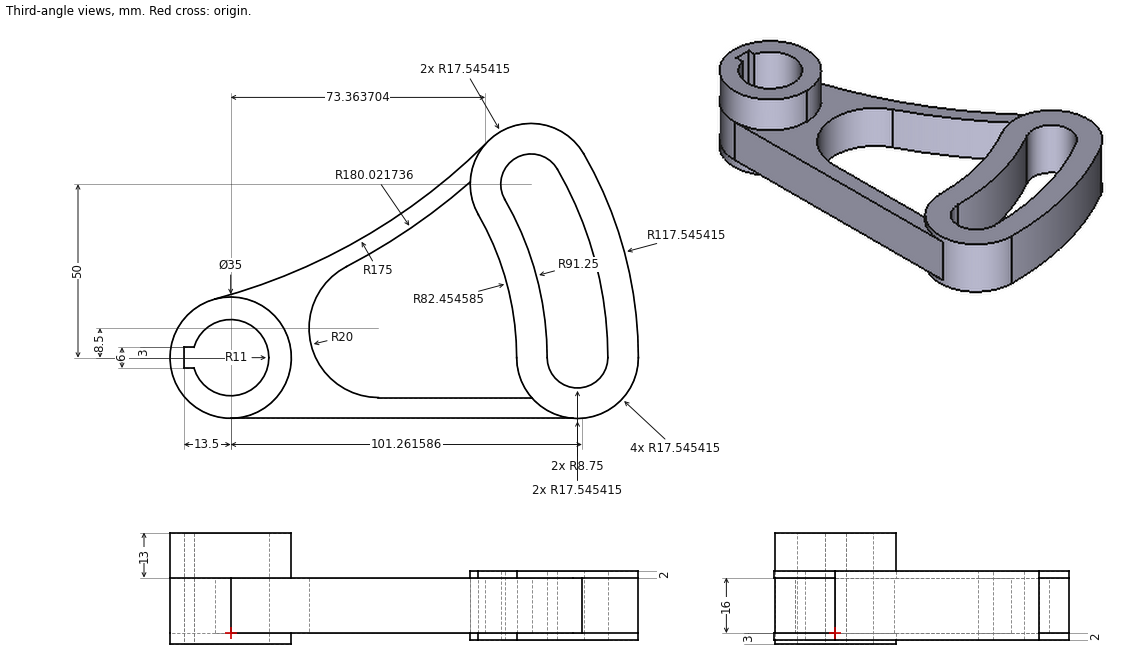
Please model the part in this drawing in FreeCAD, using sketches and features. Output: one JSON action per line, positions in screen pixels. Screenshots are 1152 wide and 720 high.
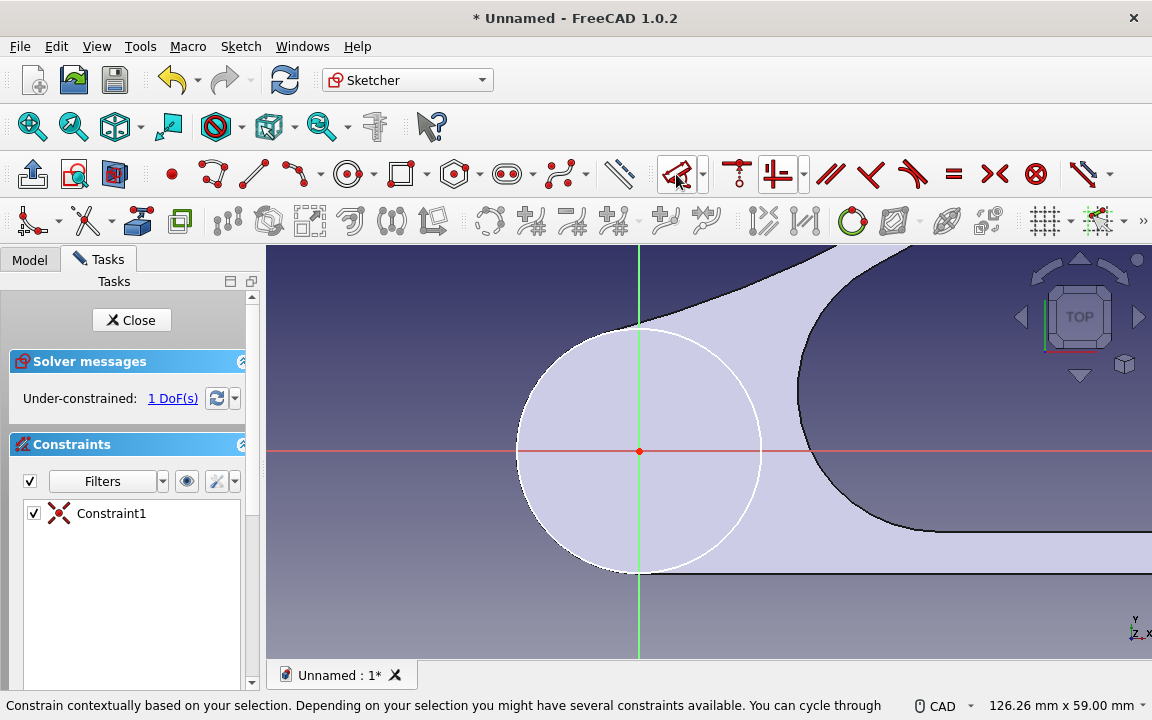
{"action": "left_click", "coordinate": [725, 364]}
{"action": "left_click", "coordinate": [747, 341]}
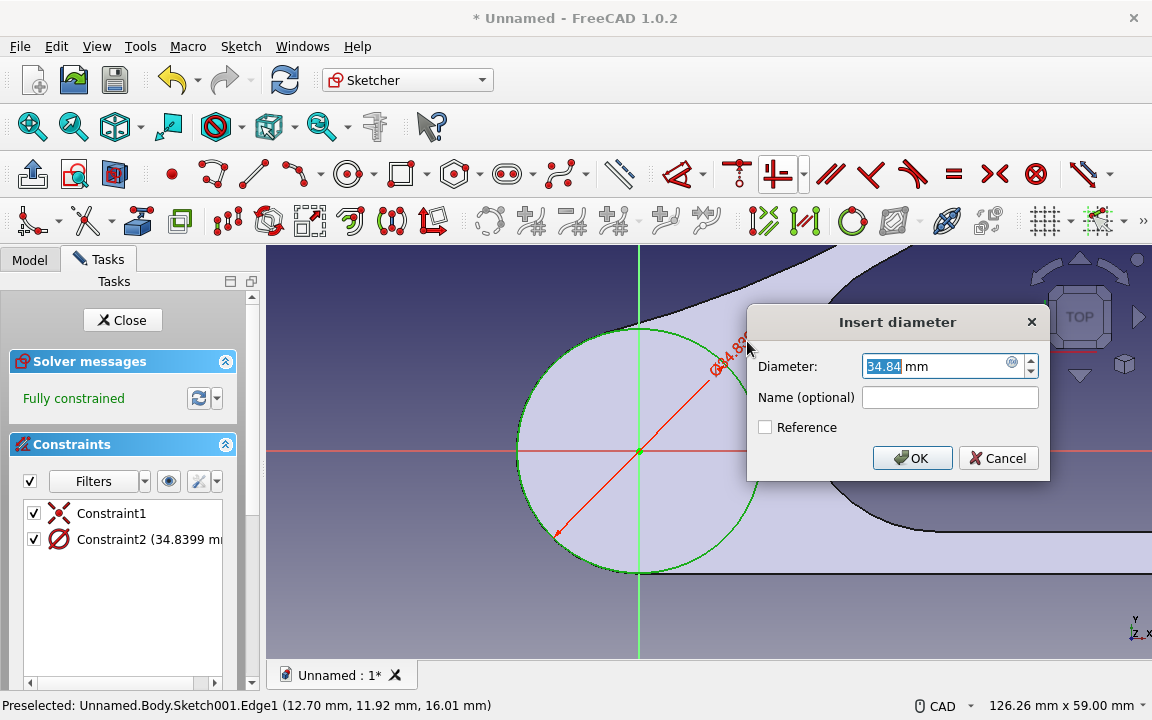
{"action": "type", "text": "35"}
{"action": "key", "text": "Return"}
{"action": "key", "text": "Escape"}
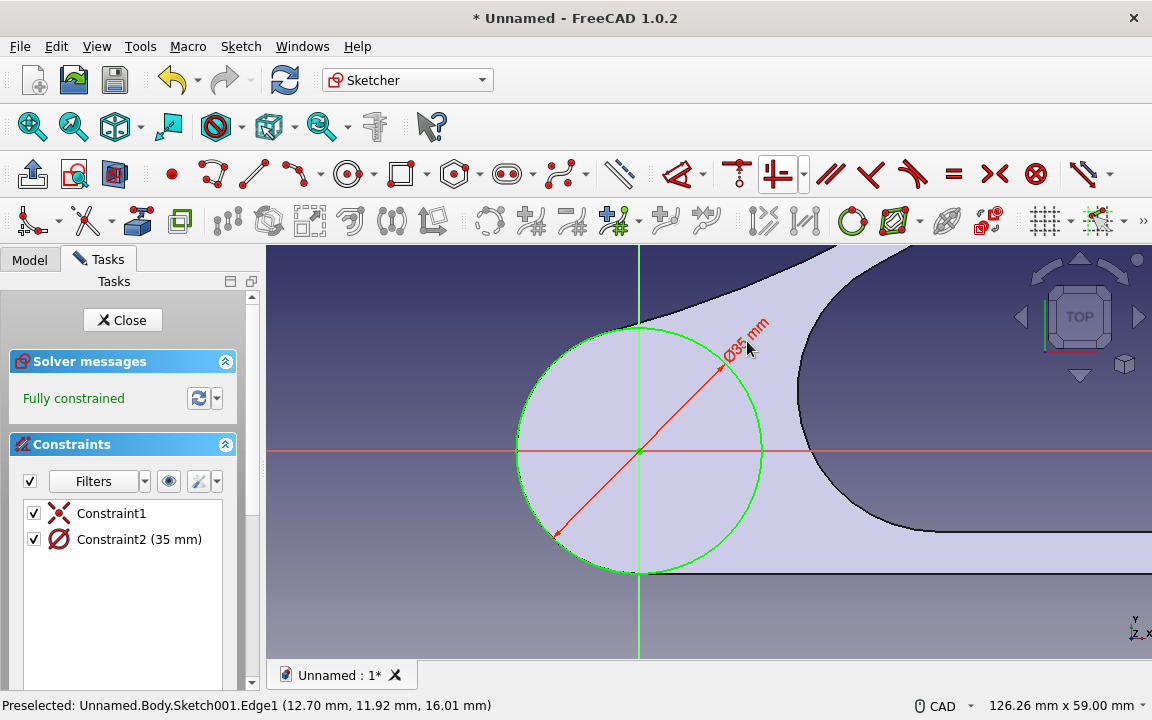
{"action": "left_click", "coordinate": [123, 320]}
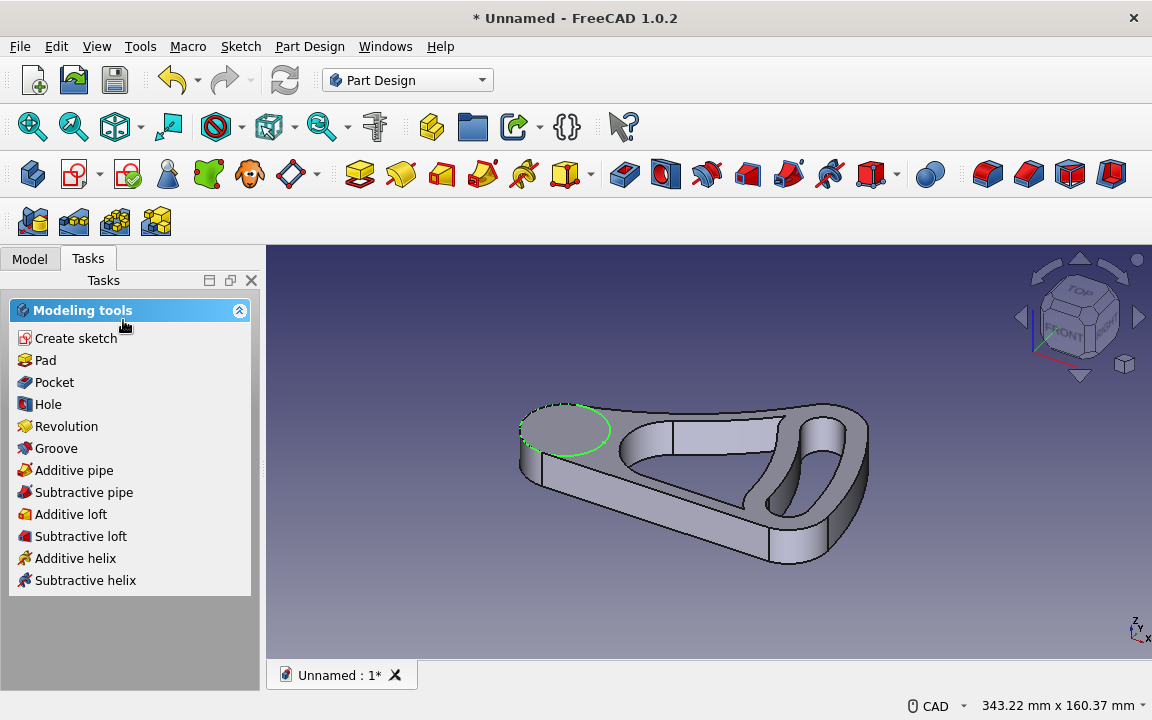
{"action": "left_click", "coordinate": [360, 174]}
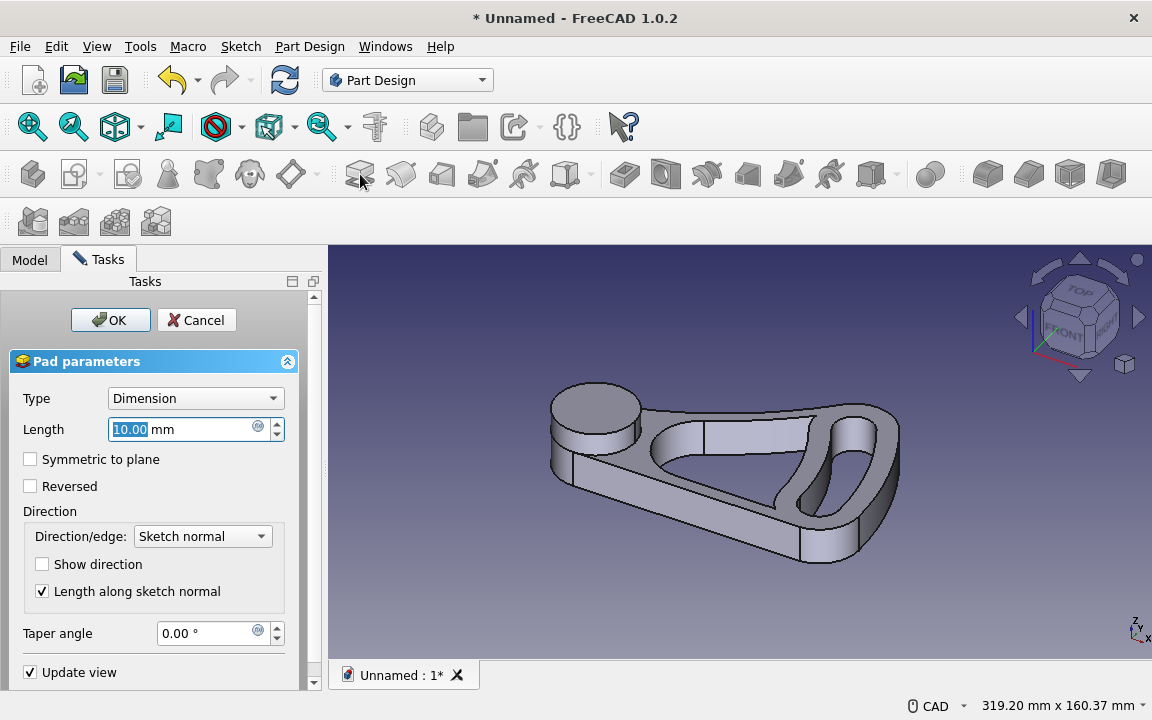
{"action": "type", "text": "13"}
{"action": "key", "text": "Tab"}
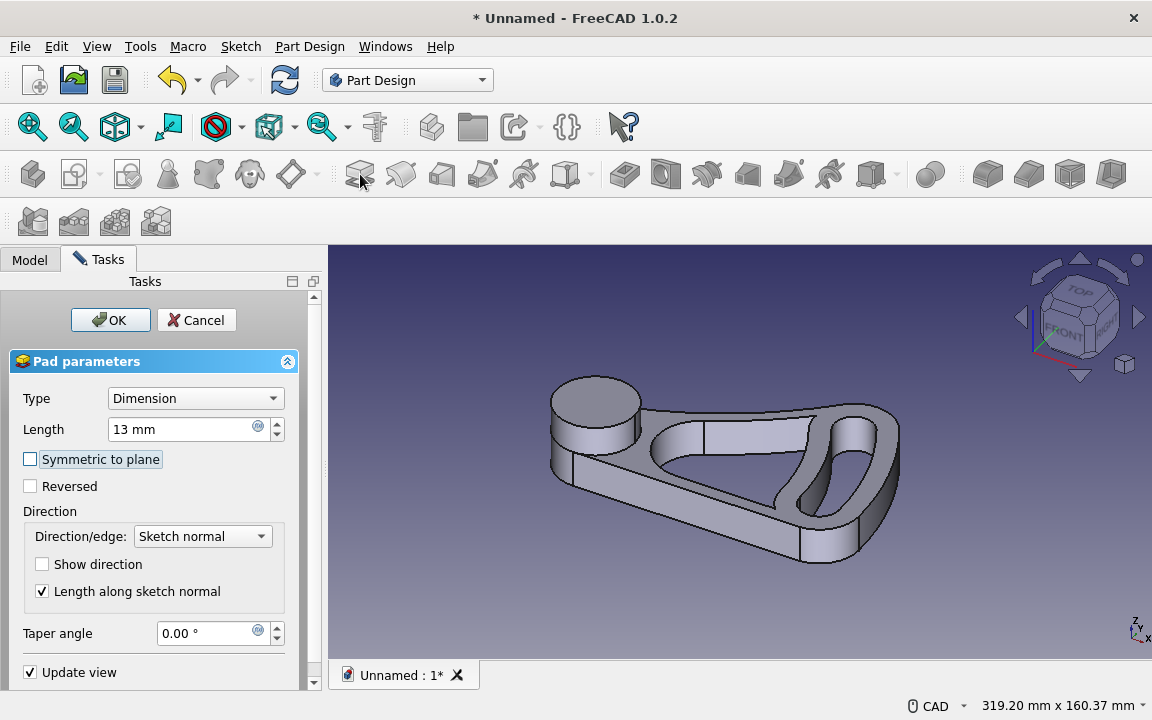
{"action": "left_click", "coordinate": [111, 320]}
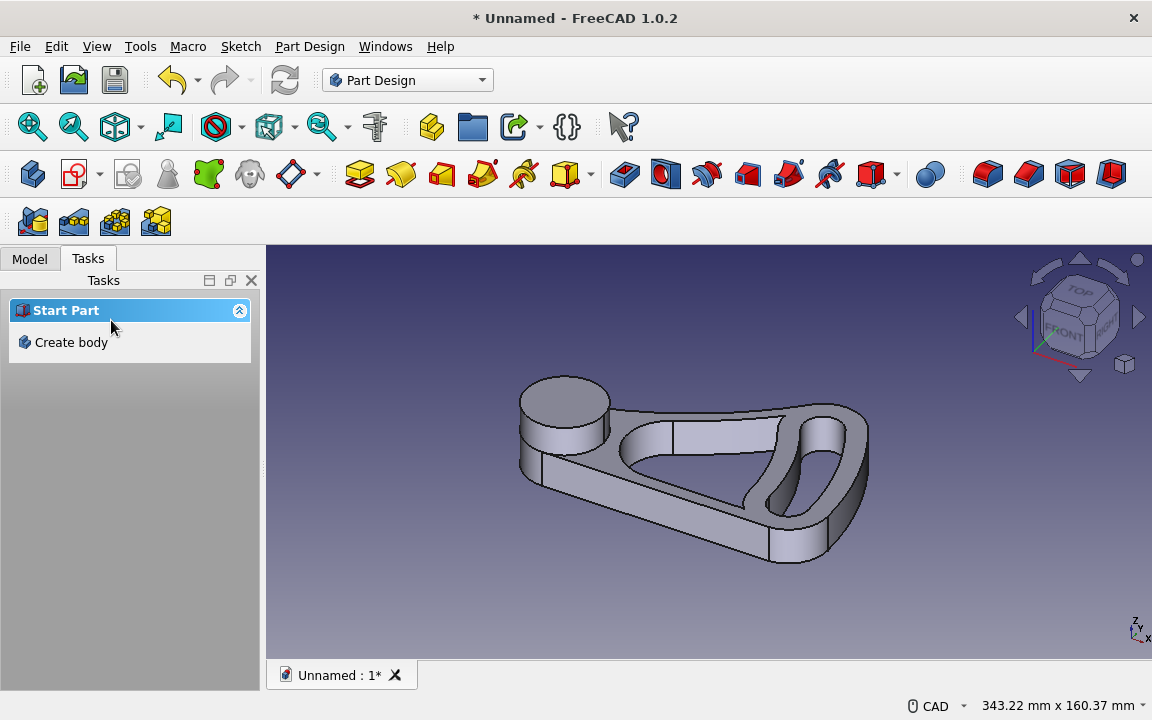
{"action": "left_click", "coordinate": [30, 258]}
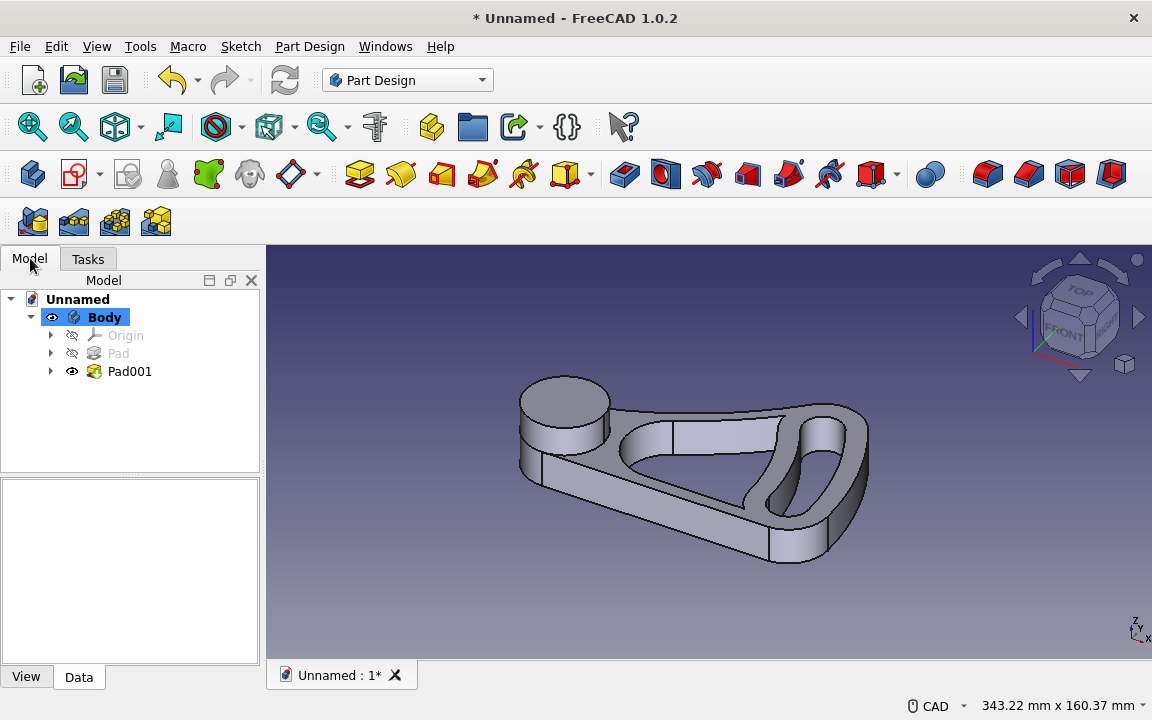
{"action": "left_click", "coordinate": [51, 335]}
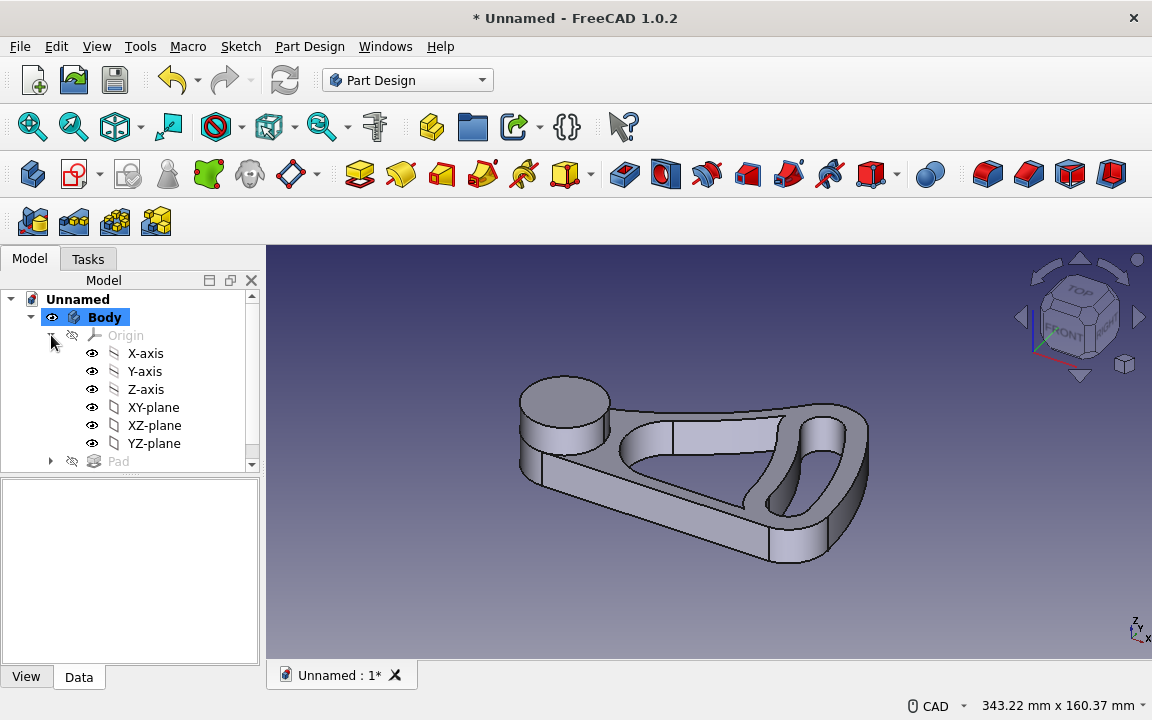
{"action": "left_click", "coordinate": [137, 407]}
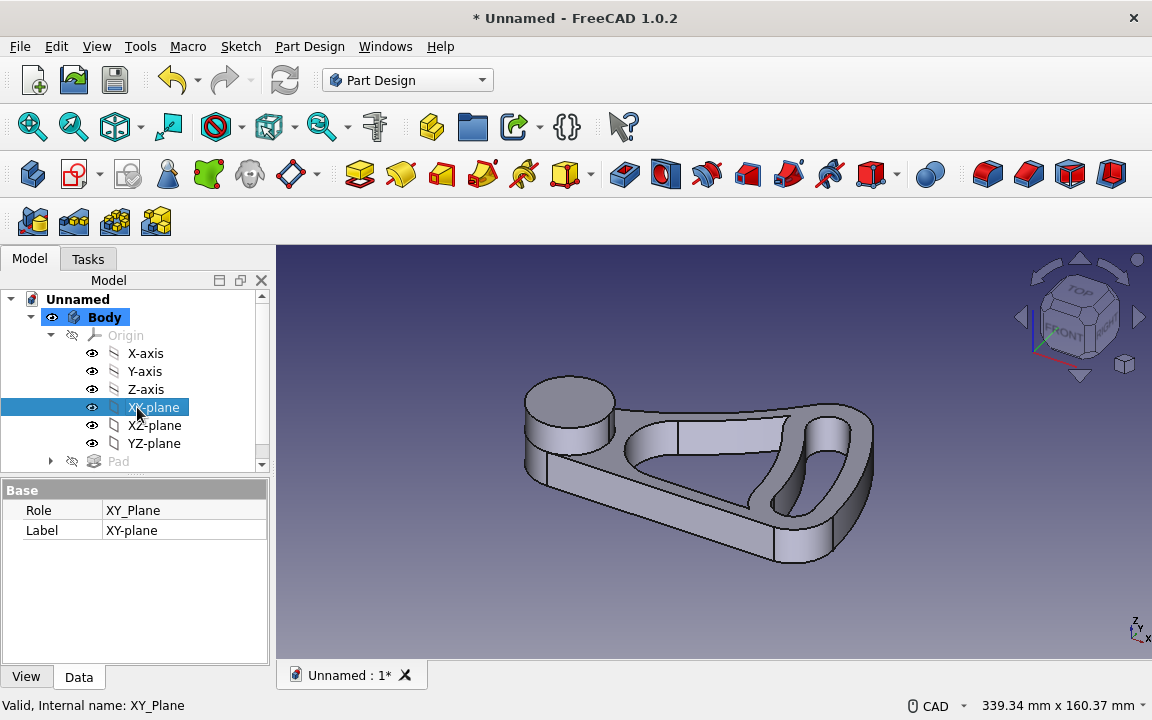
{"action": "left_click", "coordinate": [290, 174]}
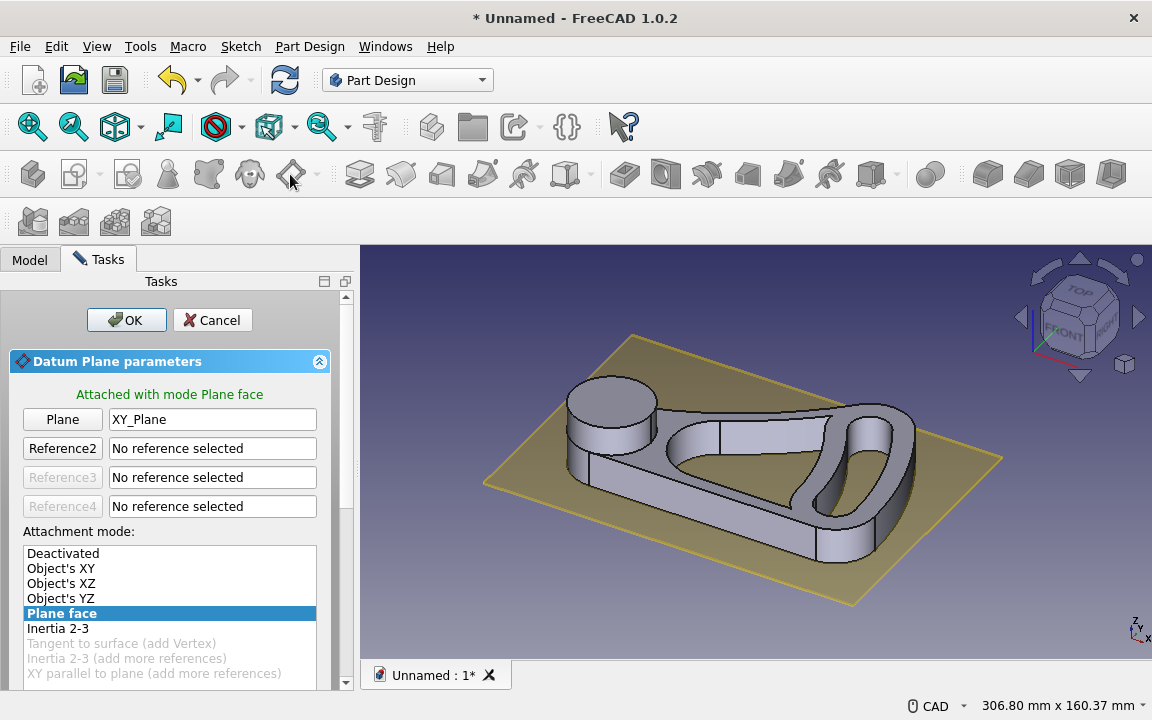
{"action": "scroll", "coordinate": [346, 490], "scroll_direction": "down", "scroll_amount": 4}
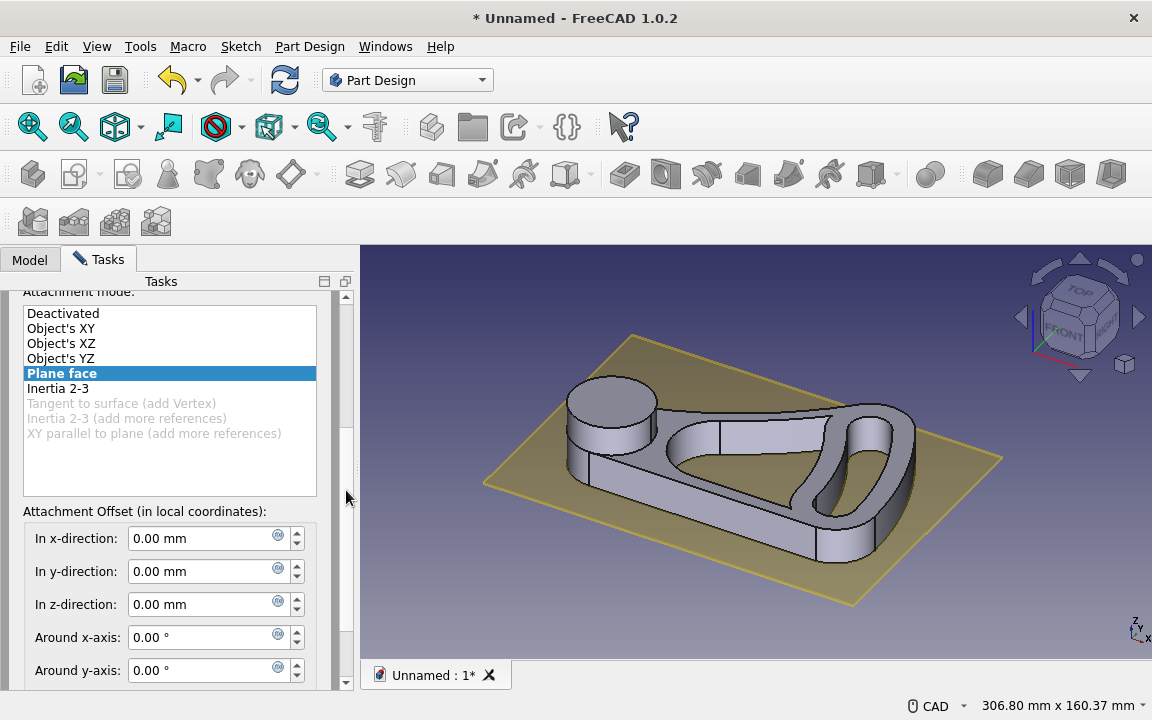
{"action": "triple_click", "coordinate": [210, 604]}